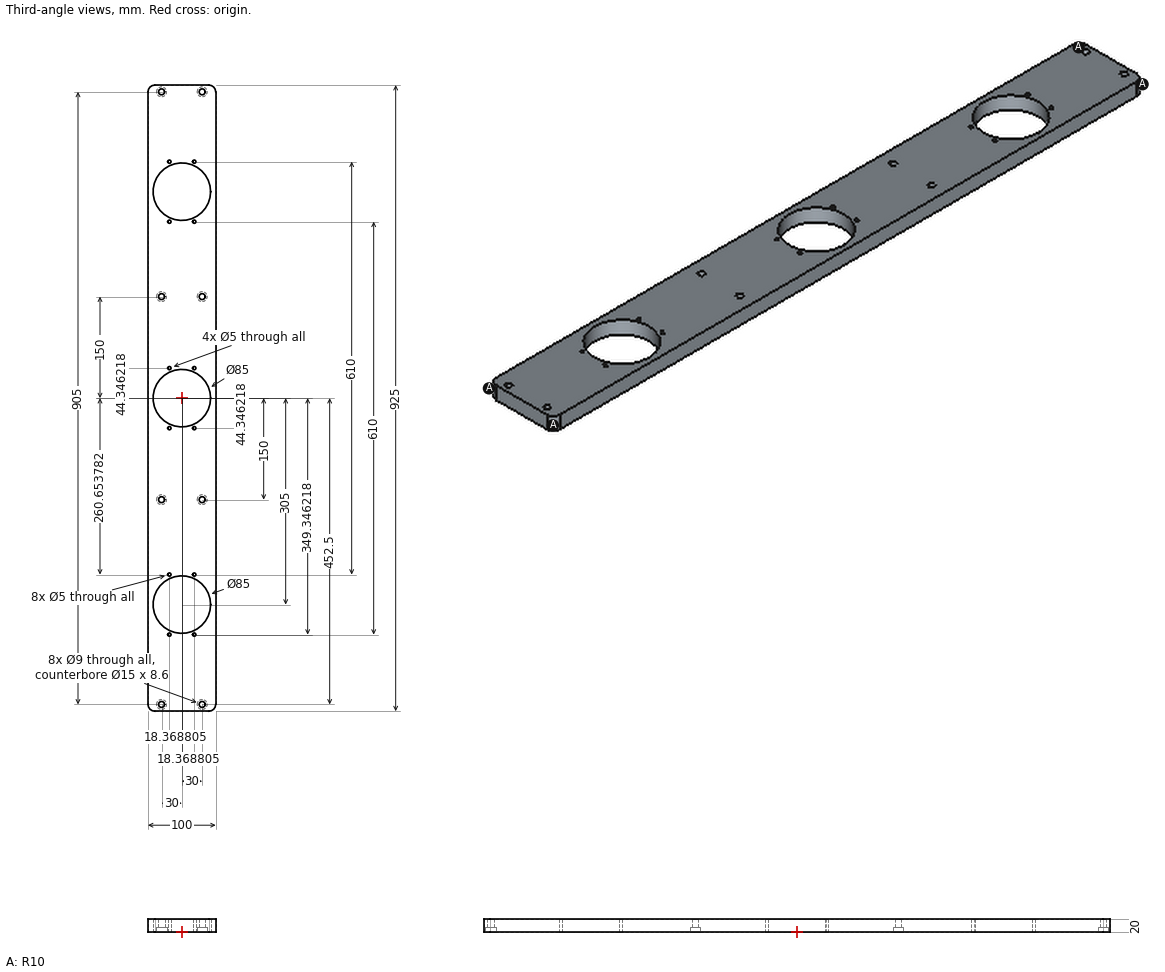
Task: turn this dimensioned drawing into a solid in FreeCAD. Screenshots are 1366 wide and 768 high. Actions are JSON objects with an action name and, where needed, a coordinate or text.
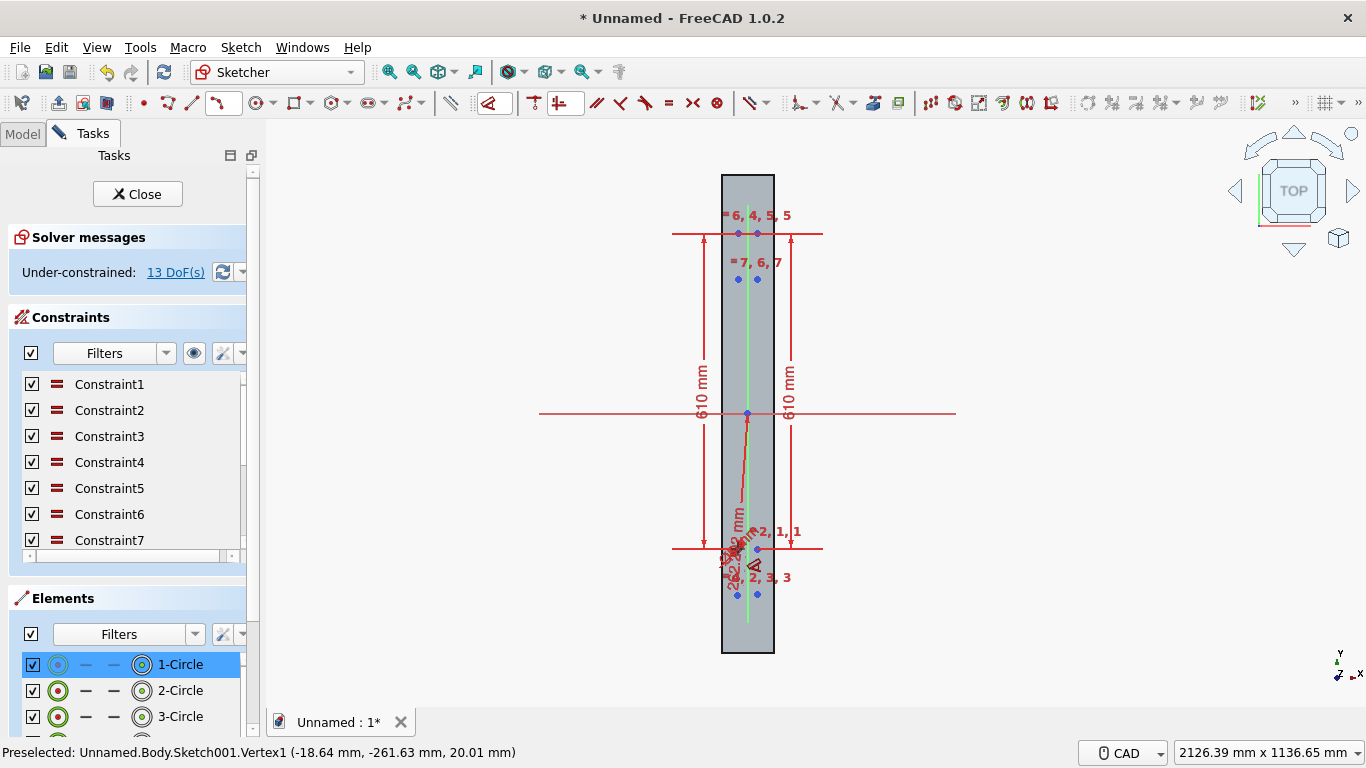
{"action": "left_click", "coordinate": [738, 233]}
{"action": "left_click", "coordinate": [704, 319]}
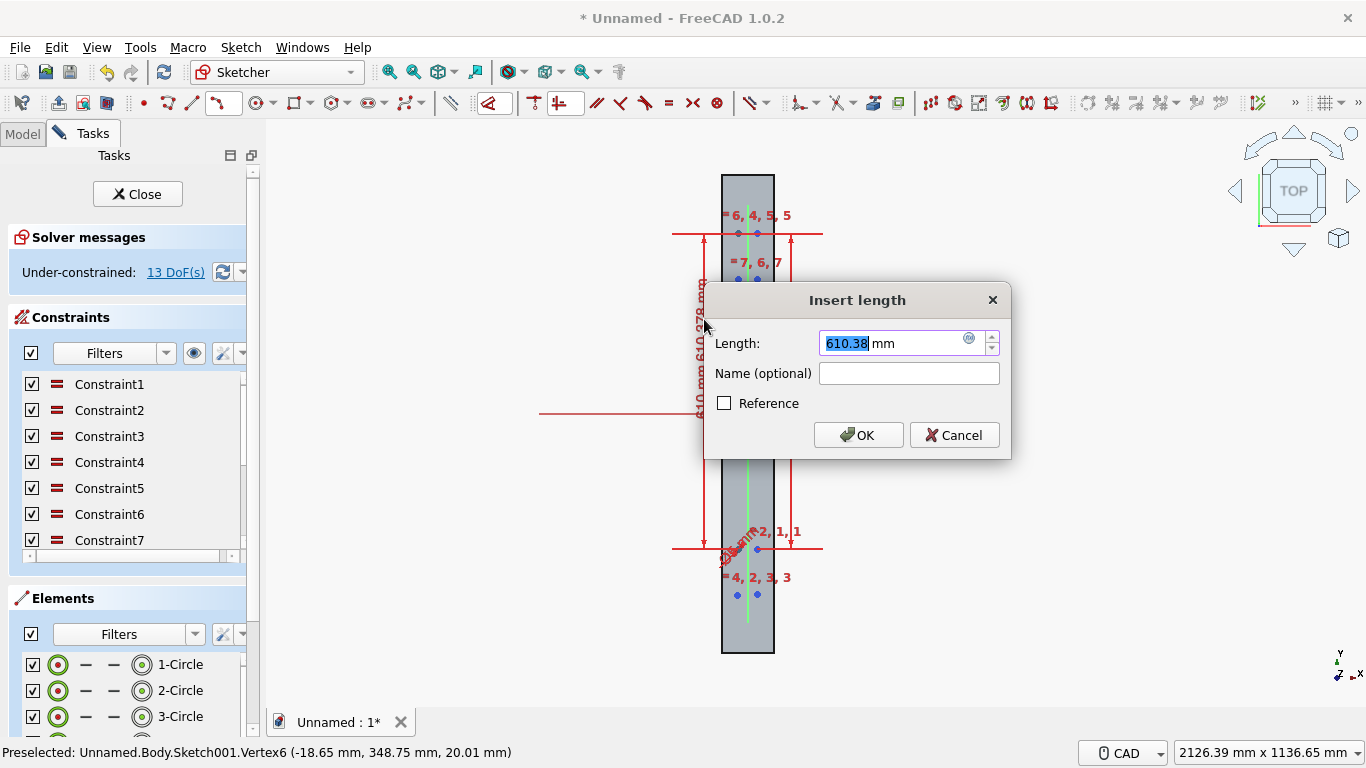
{"action": "type", "text": "610"}
{"action": "key", "text": "Return"}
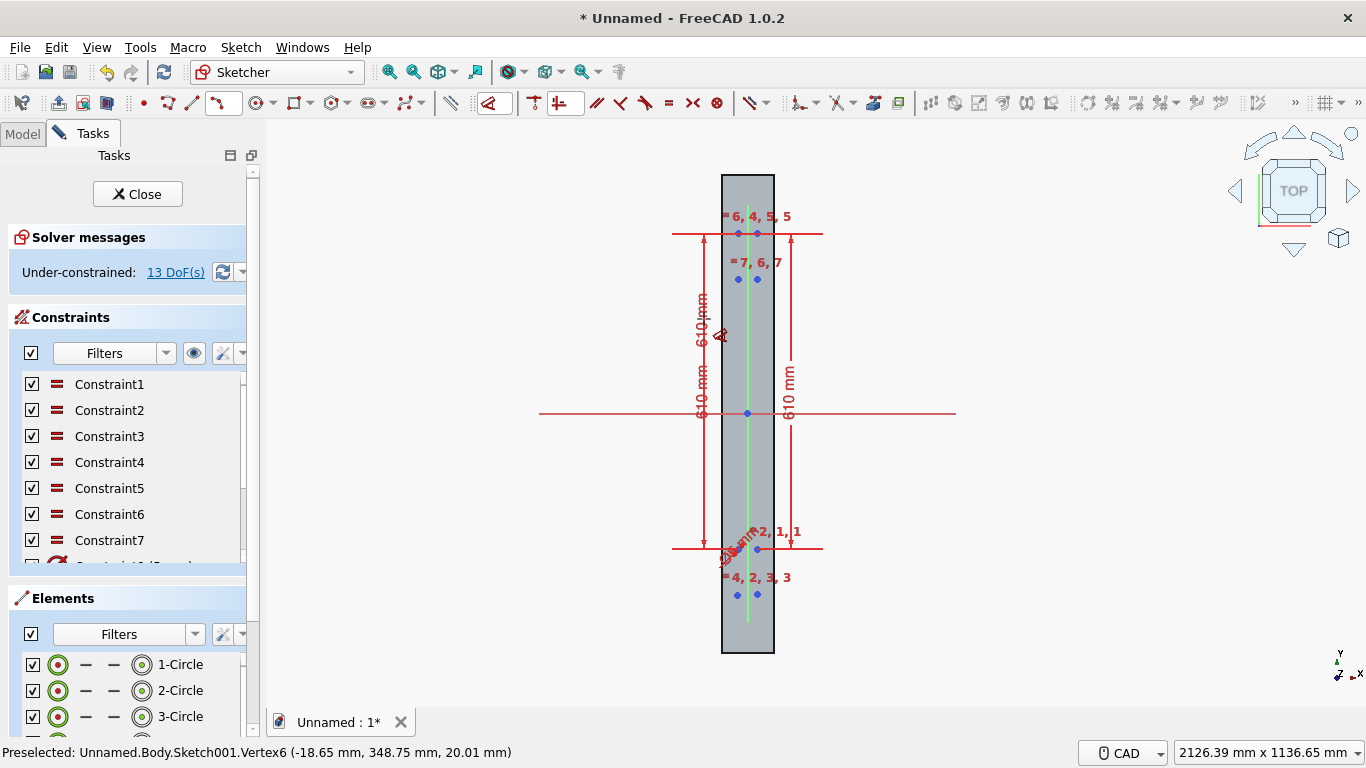
{"action": "left_click", "coordinate": [757, 595]}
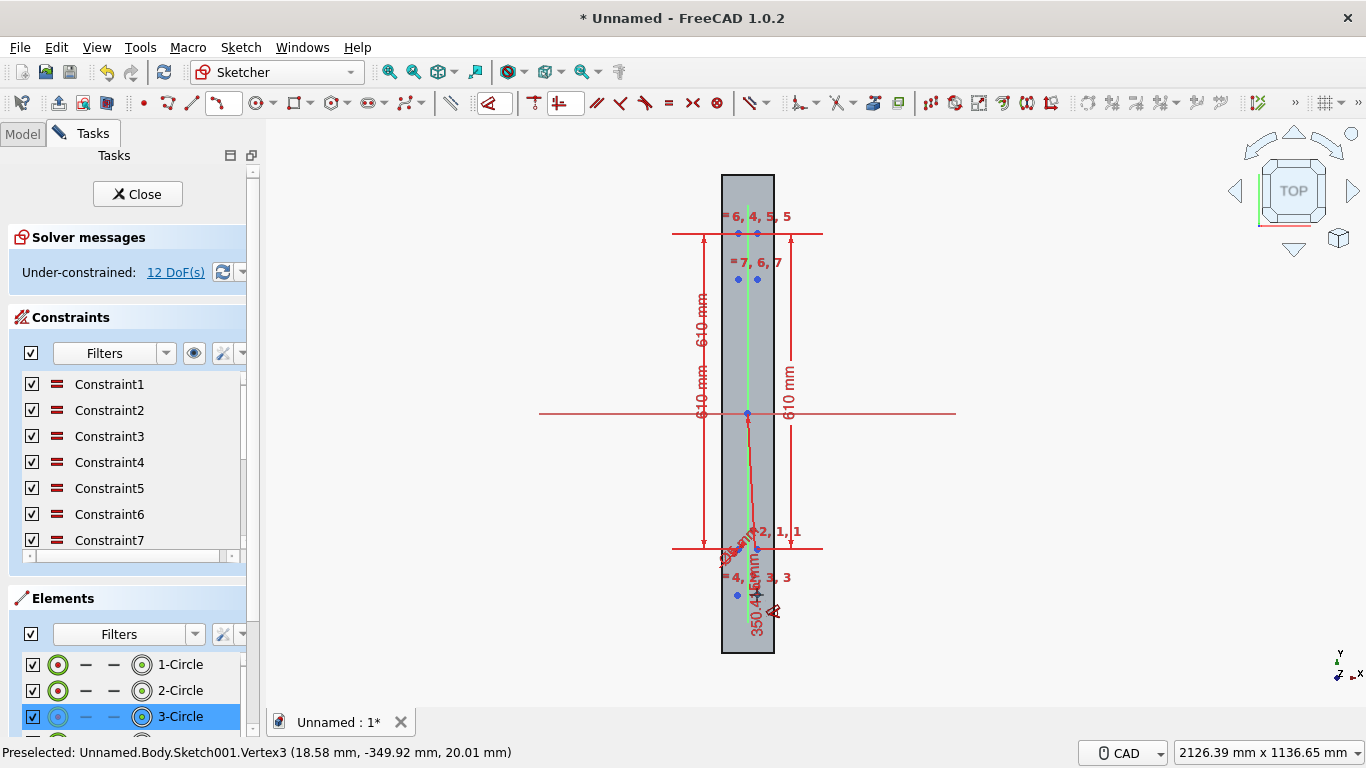
{"action": "left_click", "coordinate": [757, 280]}
{"action": "left_click", "coordinate": [791, 437]}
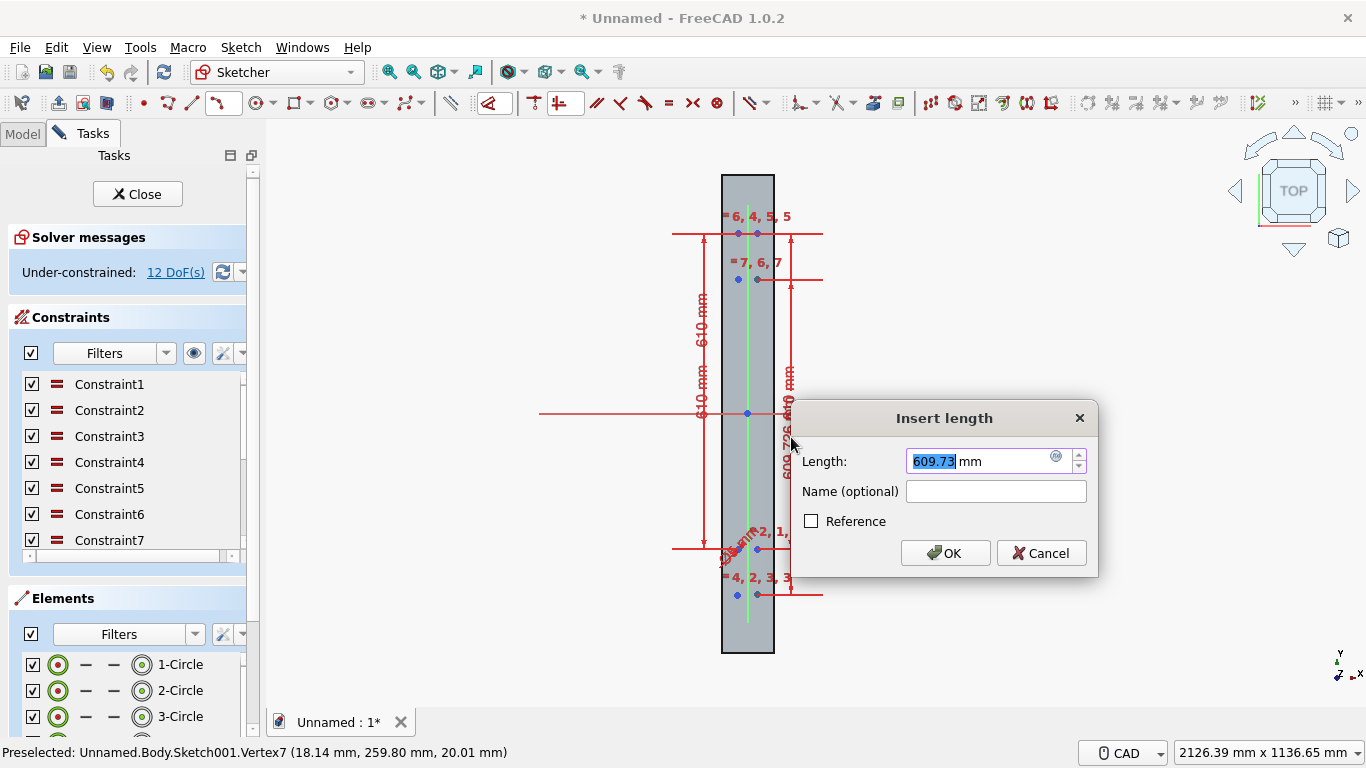
{"action": "type", "text": "610"}
{"action": "key", "text": "Return"}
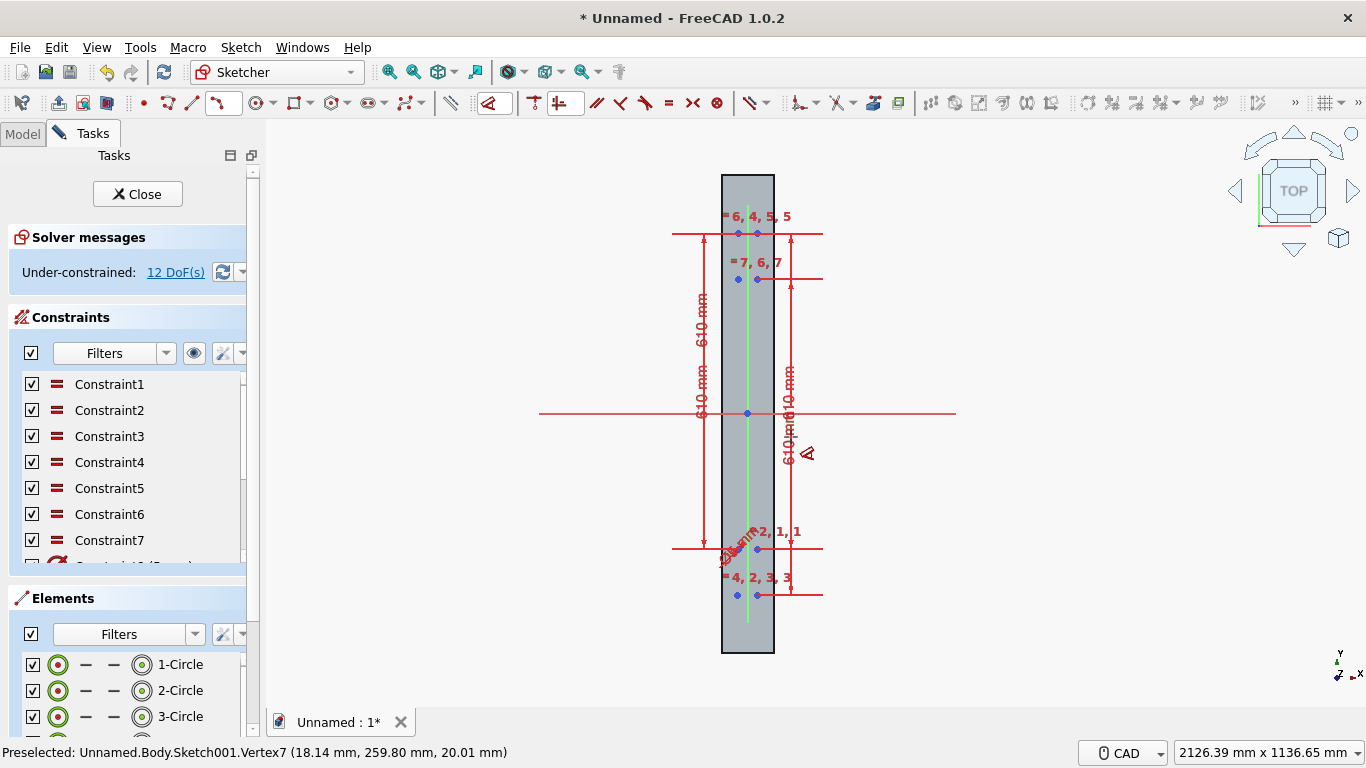
{"action": "left_click", "coordinate": [738, 595]}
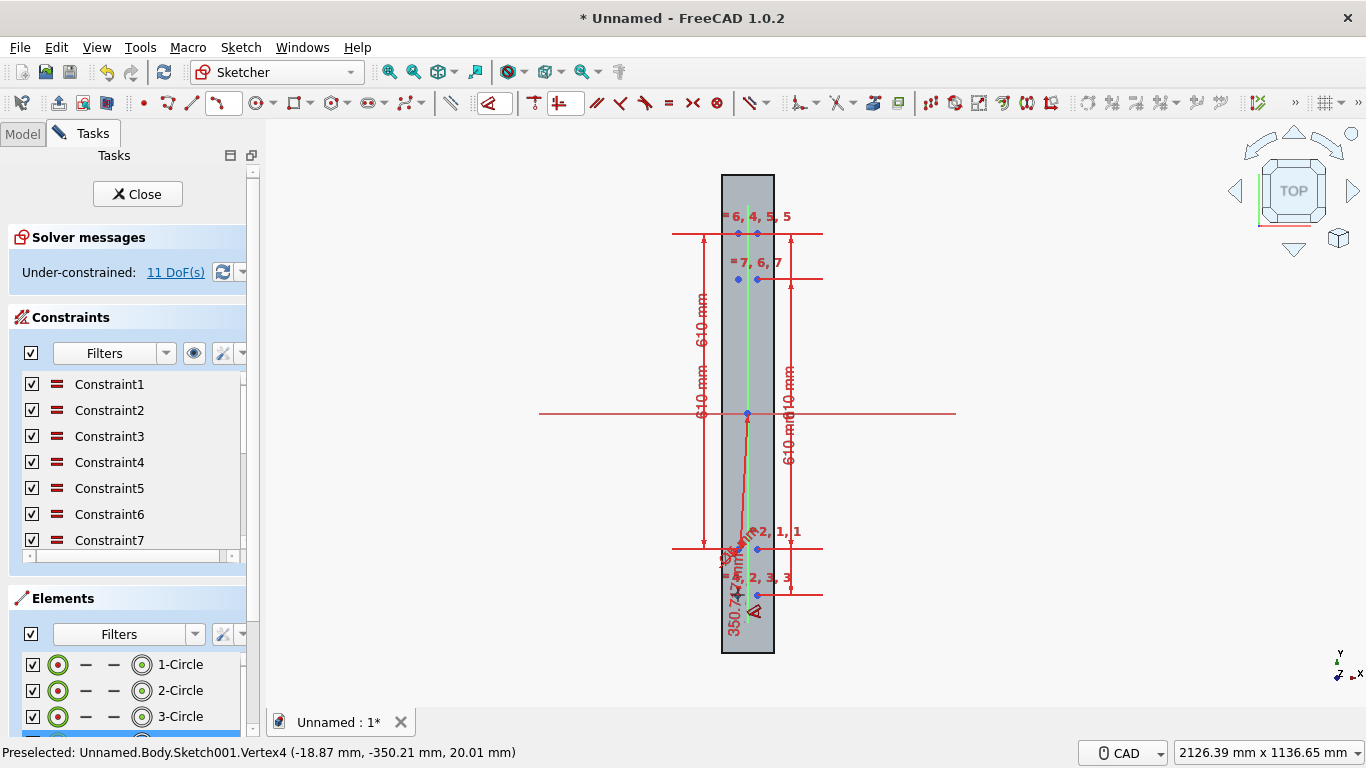
{"action": "left_click", "coordinate": [757, 279]}
{"action": "left_click", "coordinate": [704, 437]}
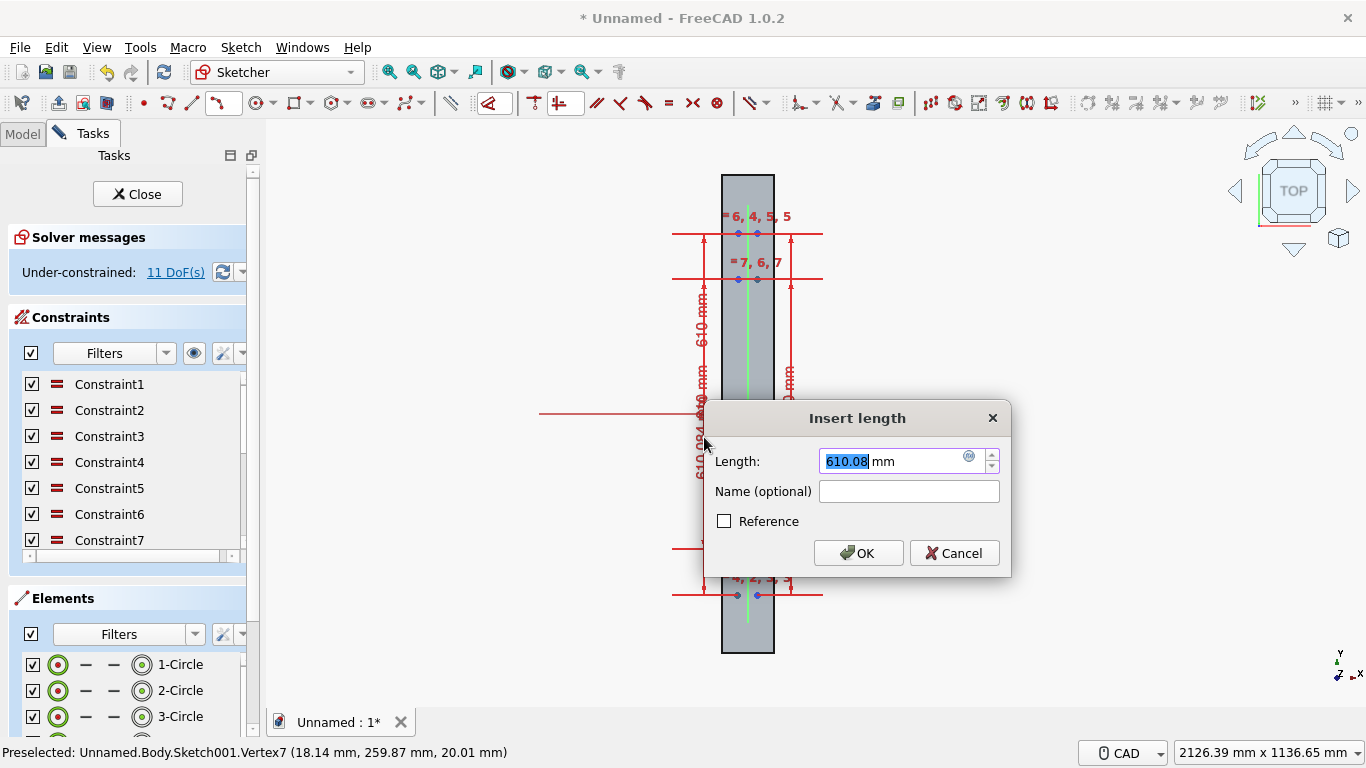
{"action": "type", "text": "610"}
{"action": "key", "text": "Return"}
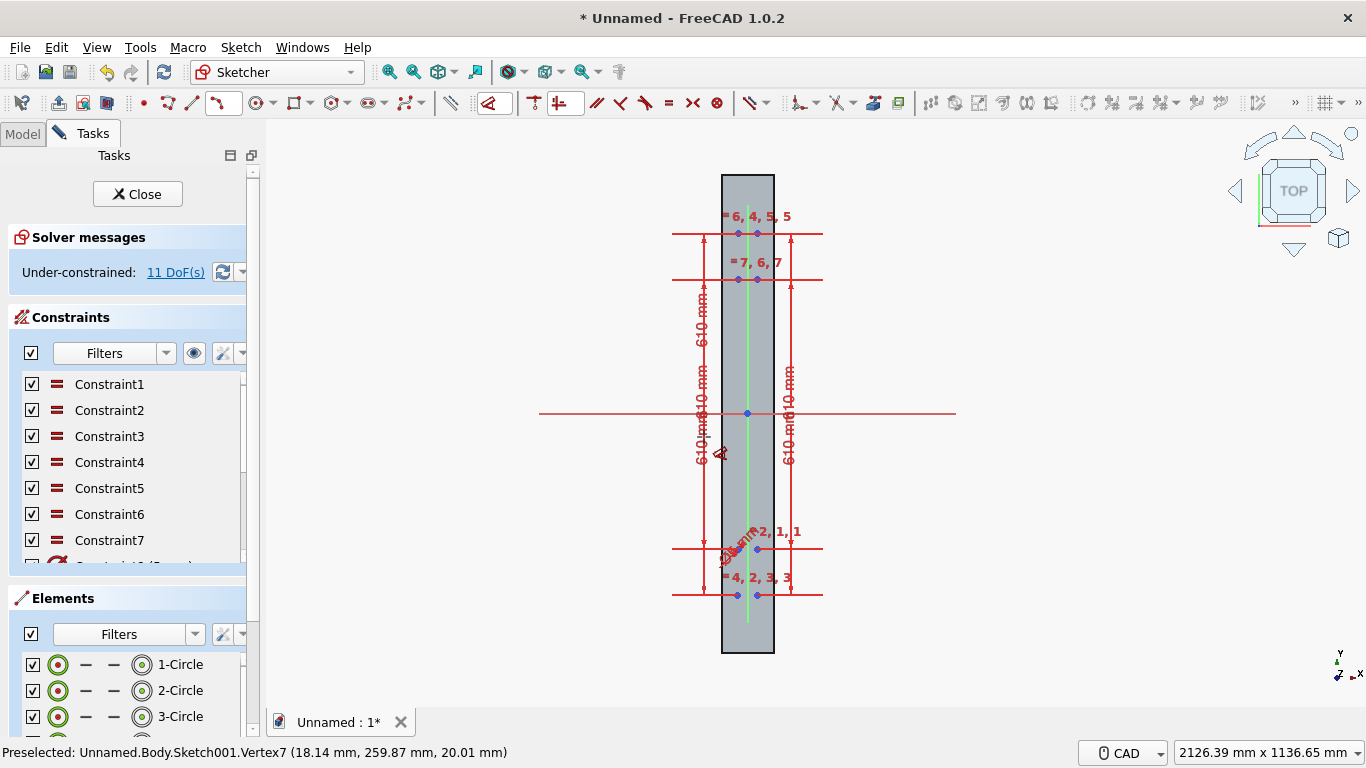
{"action": "left_click", "coordinate": [738, 595]}